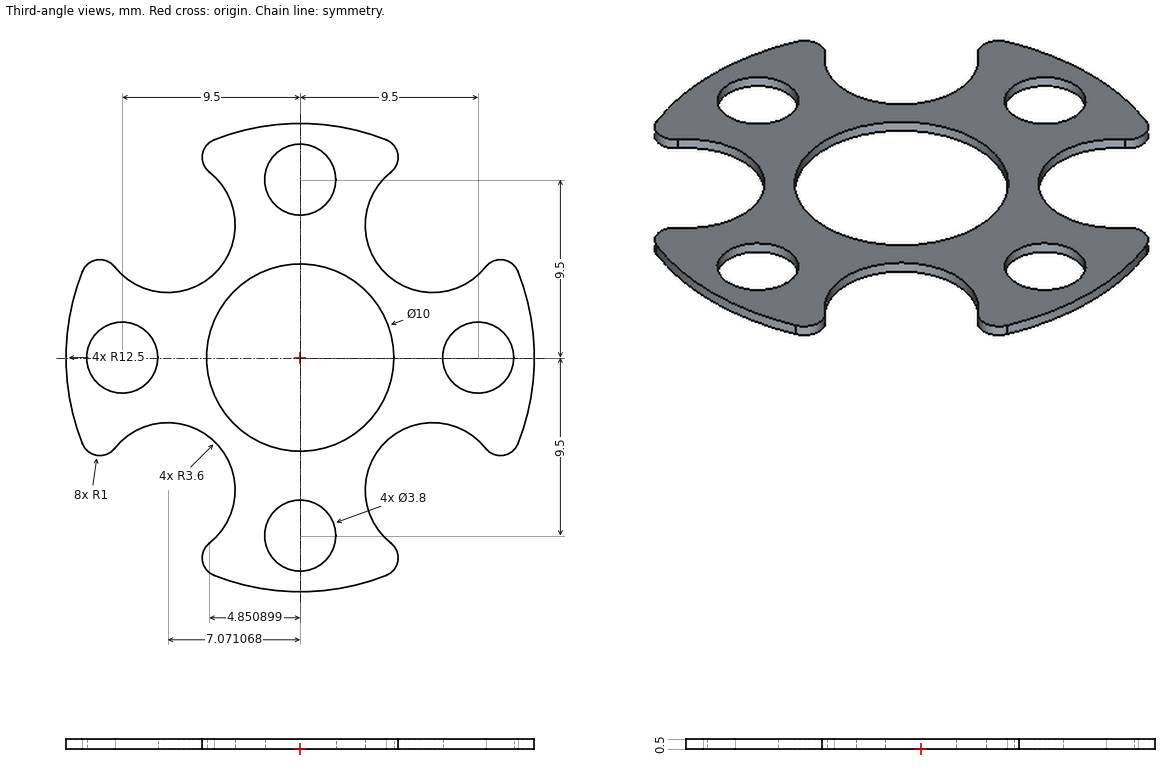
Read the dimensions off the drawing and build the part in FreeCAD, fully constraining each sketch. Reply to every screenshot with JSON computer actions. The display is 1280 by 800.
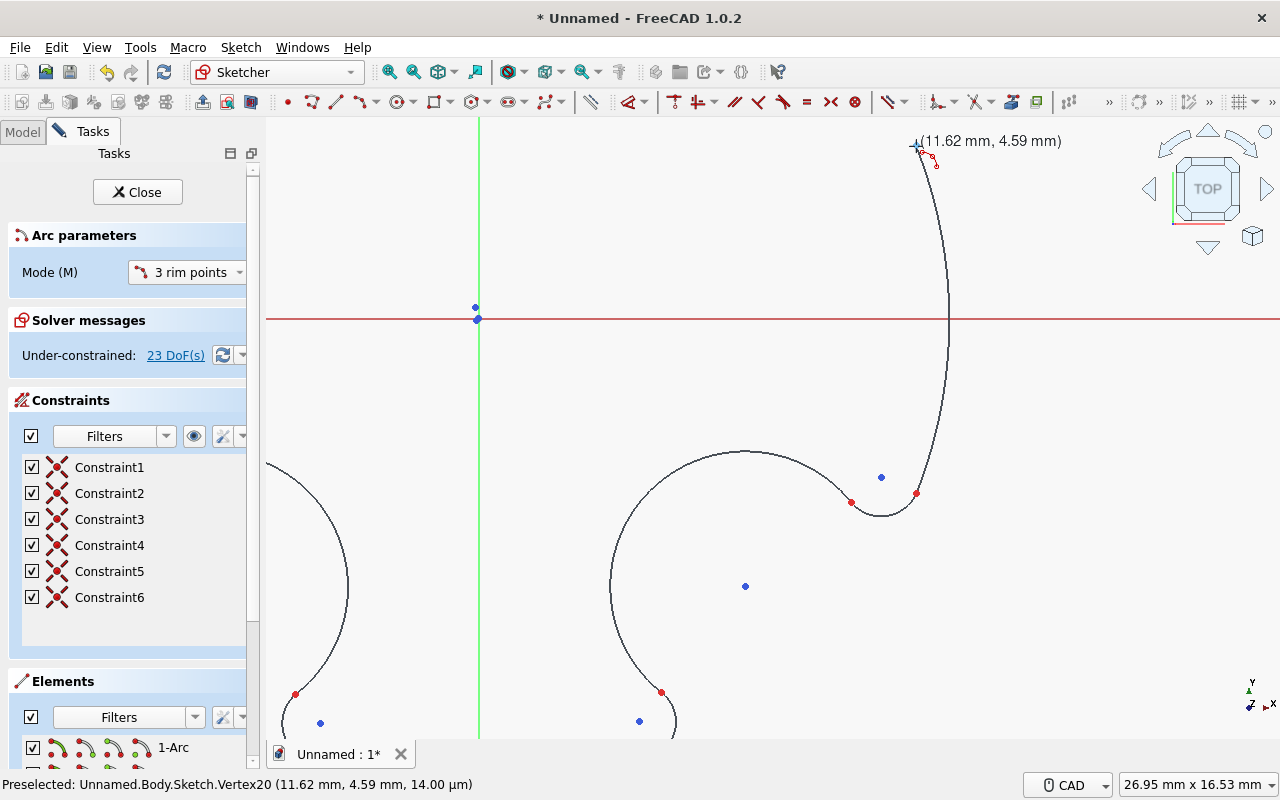
{"action": "scroll", "coordinate": [889, 517], "scroll_direction": "down", "scroll_amount": 4}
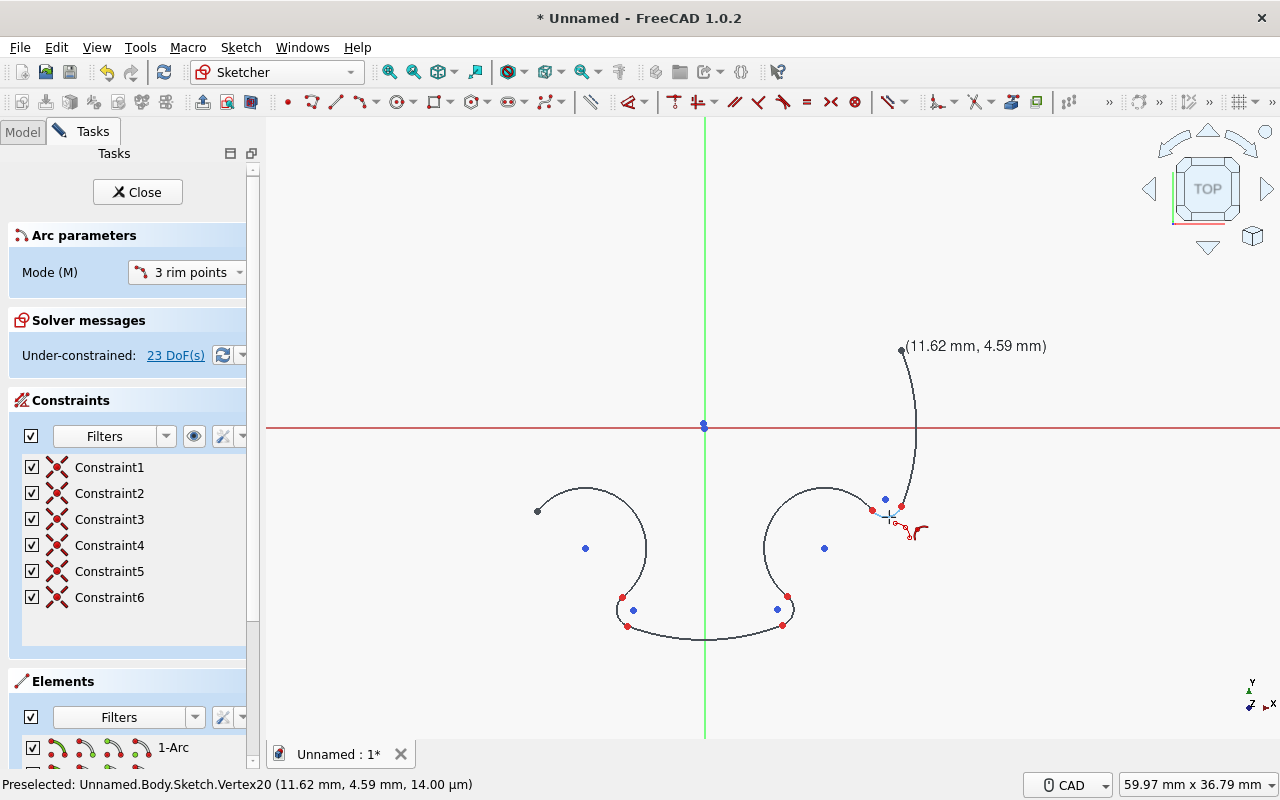
{"action": "left_click", "coordinate": [872, 346]}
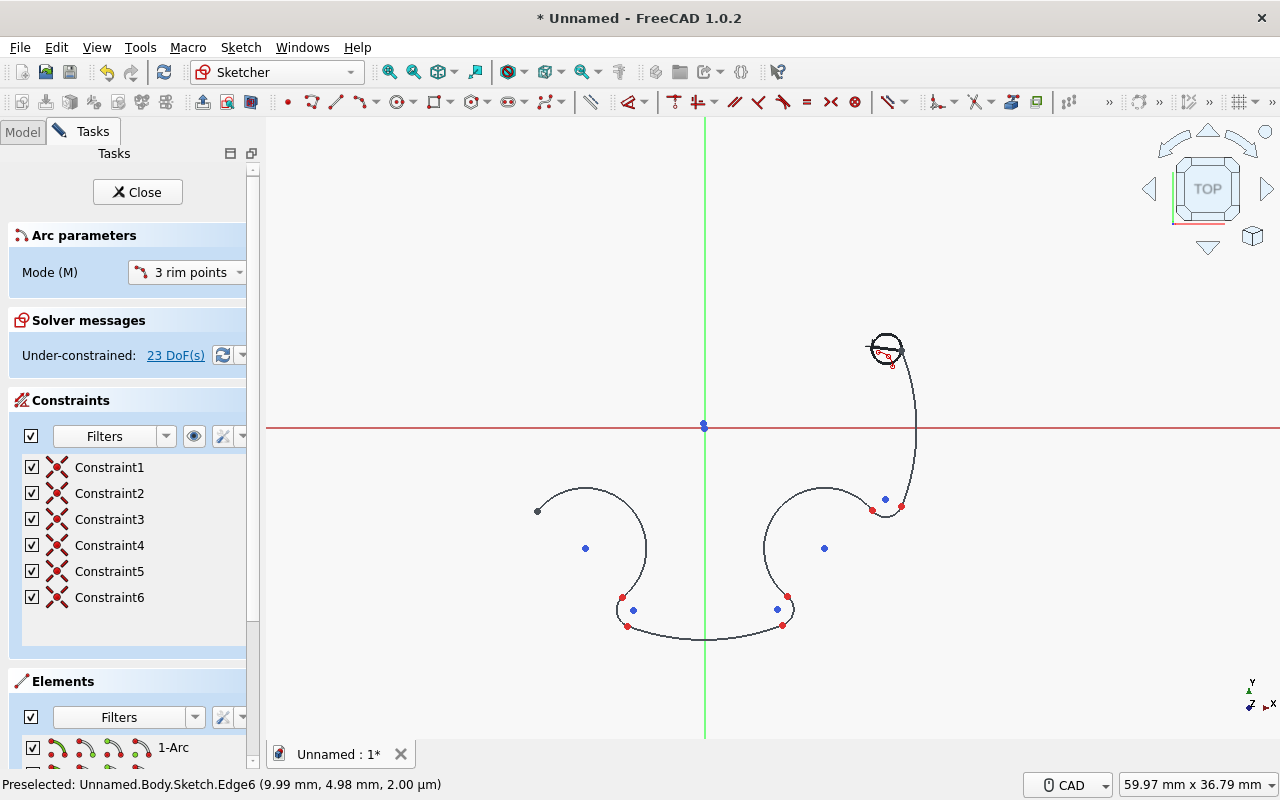
{"action": "scroll", "coordinate": [888, 340], "scroll_direction": "up", "scroll_amount": 4}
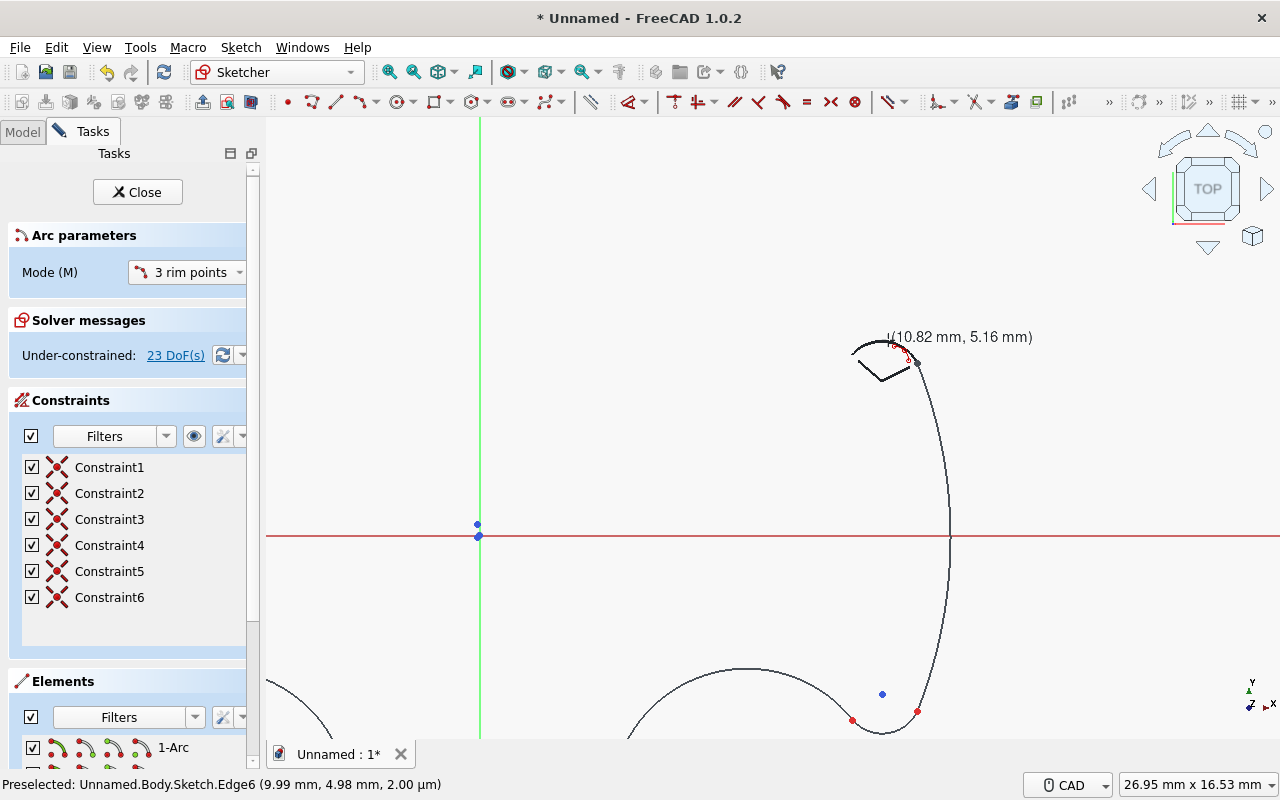
{"action": "left_click", "coordinate": [888, 339]}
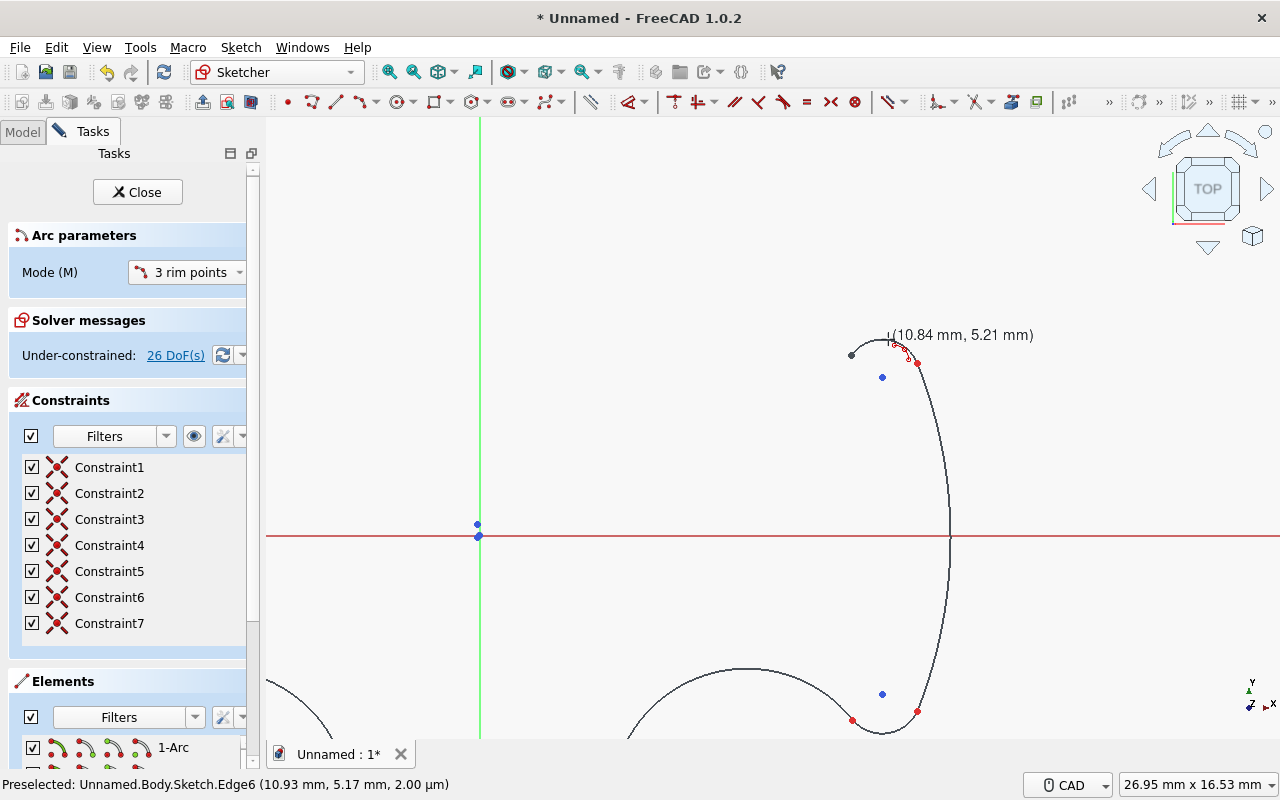
{"action": "left_click", "coordinate": [852, 355]}
{"action": "left_click", "coordinate": [662, 163]}
{"action": "left_click", "coordinate": [650, 366]}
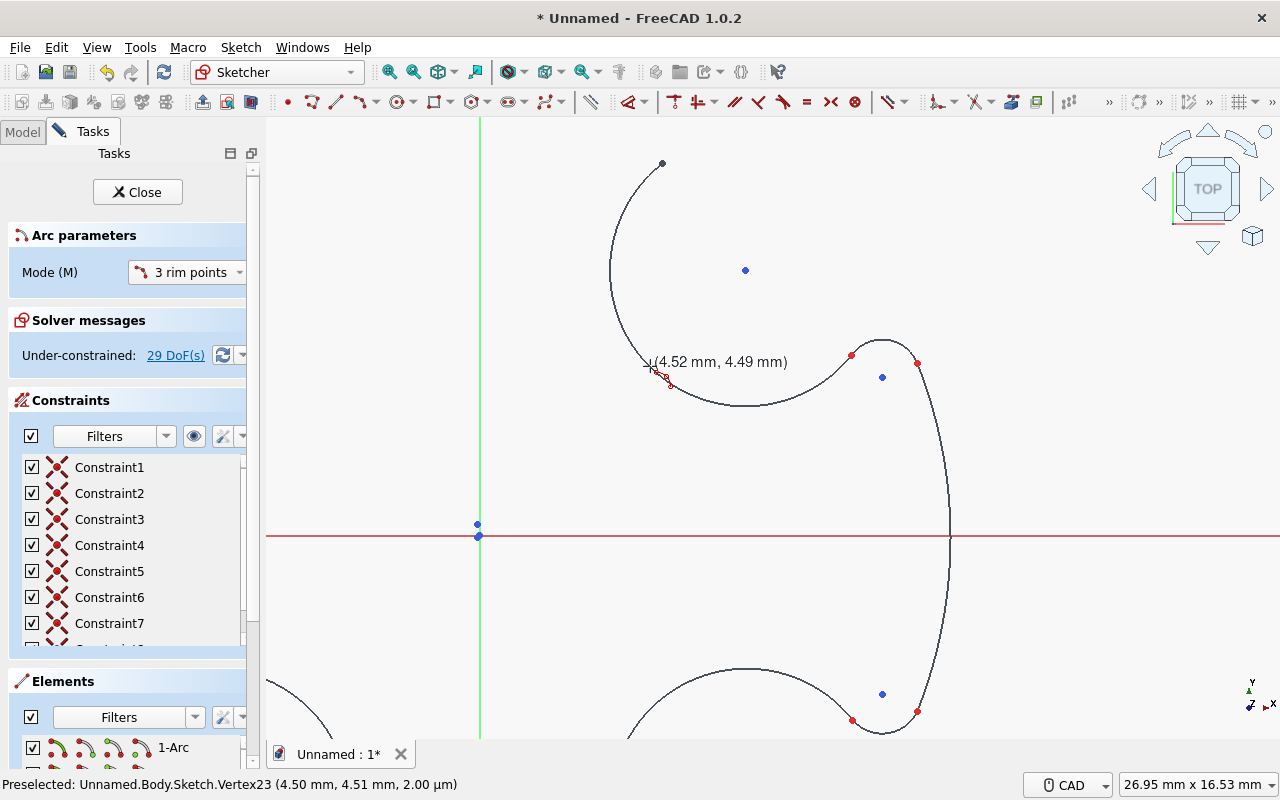
{"action": "left_click", "coordinate": [662, 164]}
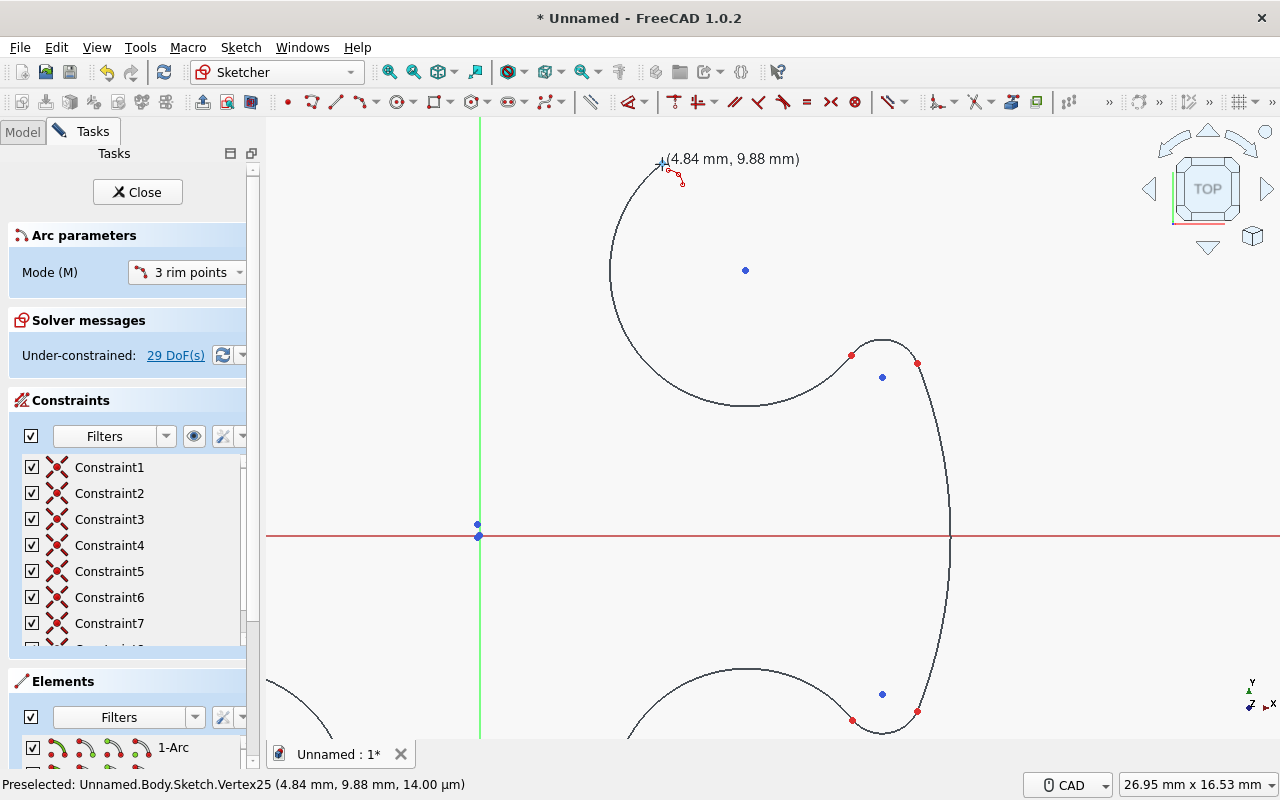
{"action": "scroll", "coordinate": [888, 340], "scroll_direction": "down", "scroll_amount": 4}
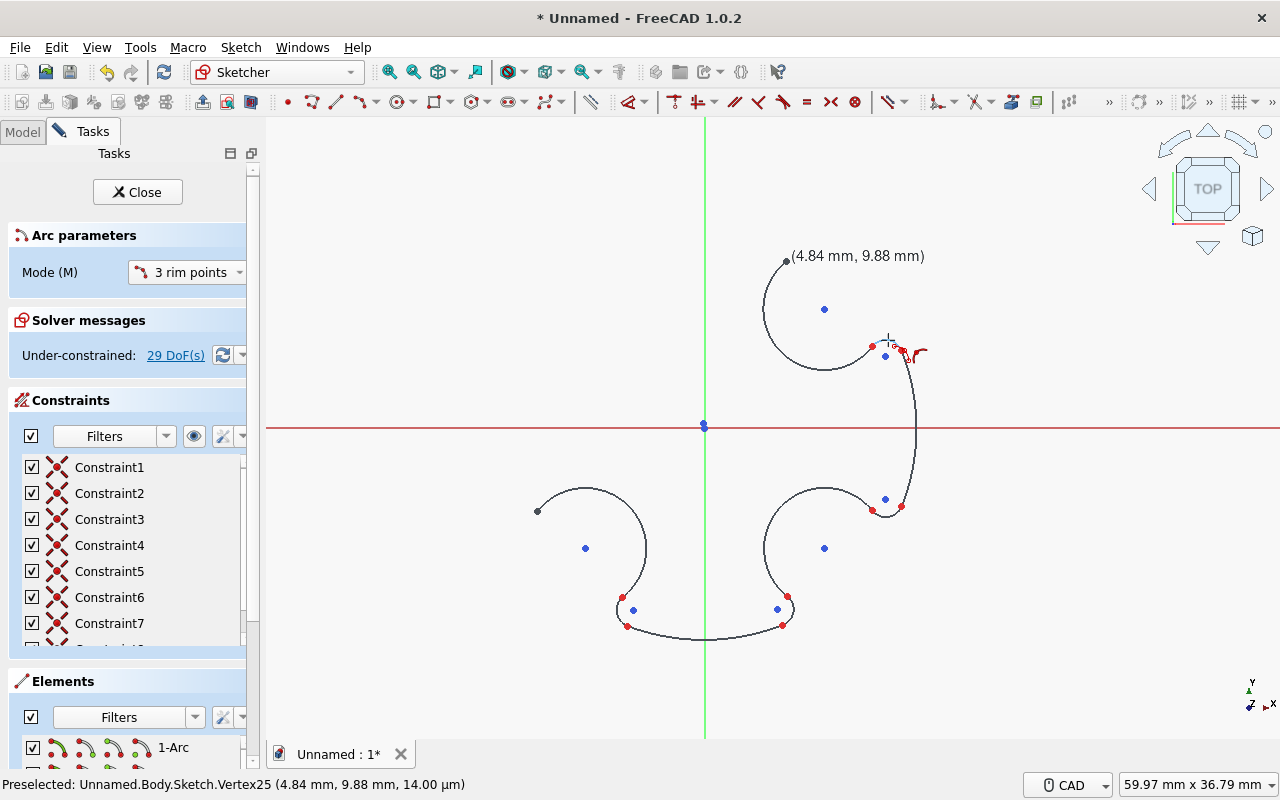
{"action": "left_click", "coordinate": [783, 232]}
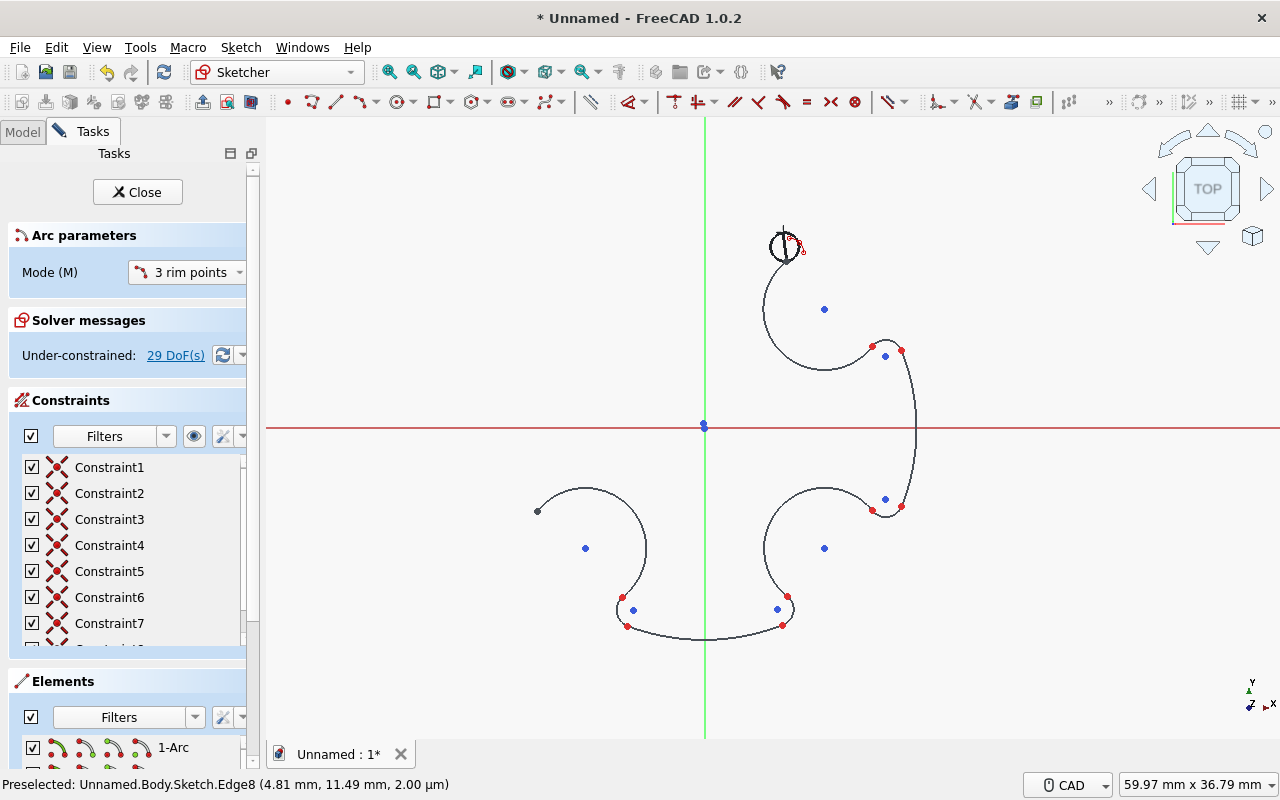
{"action": "scroll", "coordinate": [793, 245], "scroll_direction": "up", "scroll_amount": 4}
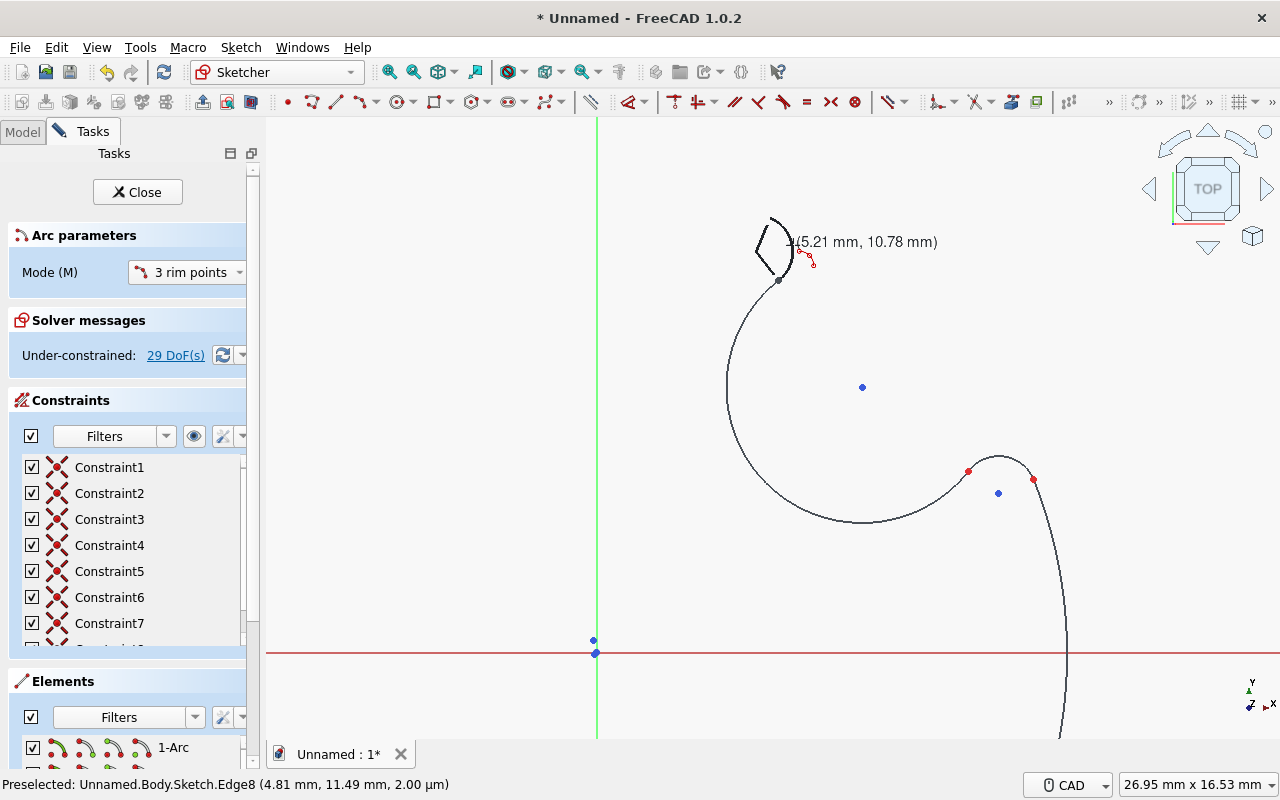
{"action": "left_click", "coordinate": [793, 245]}